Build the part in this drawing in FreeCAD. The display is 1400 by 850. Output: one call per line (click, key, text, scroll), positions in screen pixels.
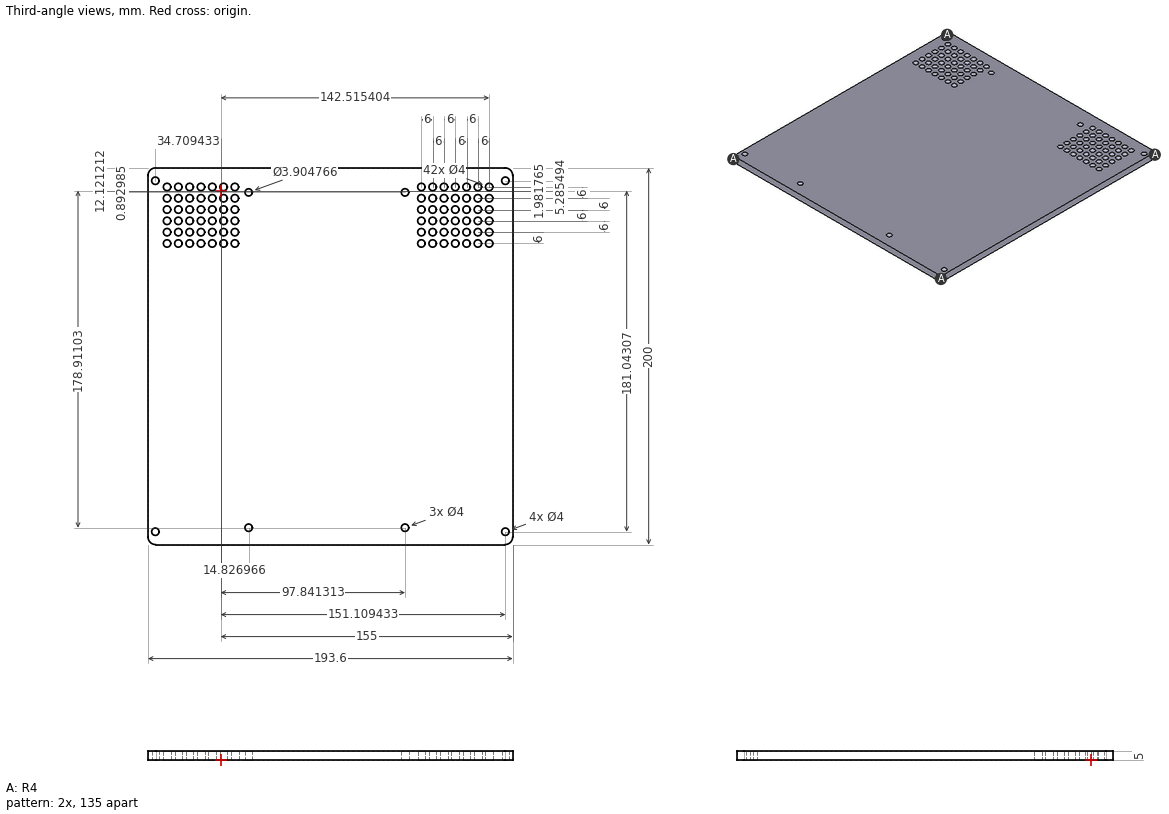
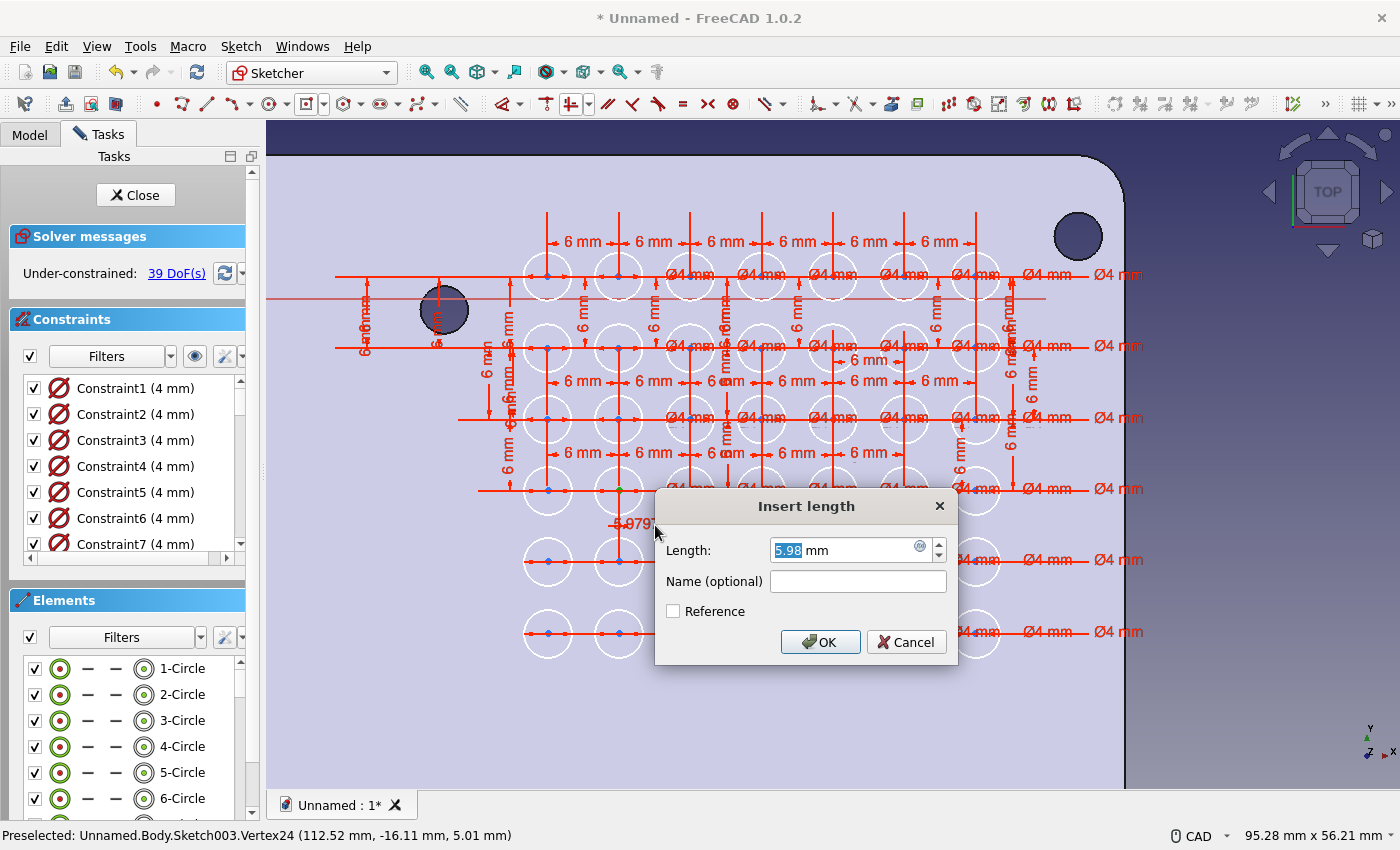
text(6)
key(Return)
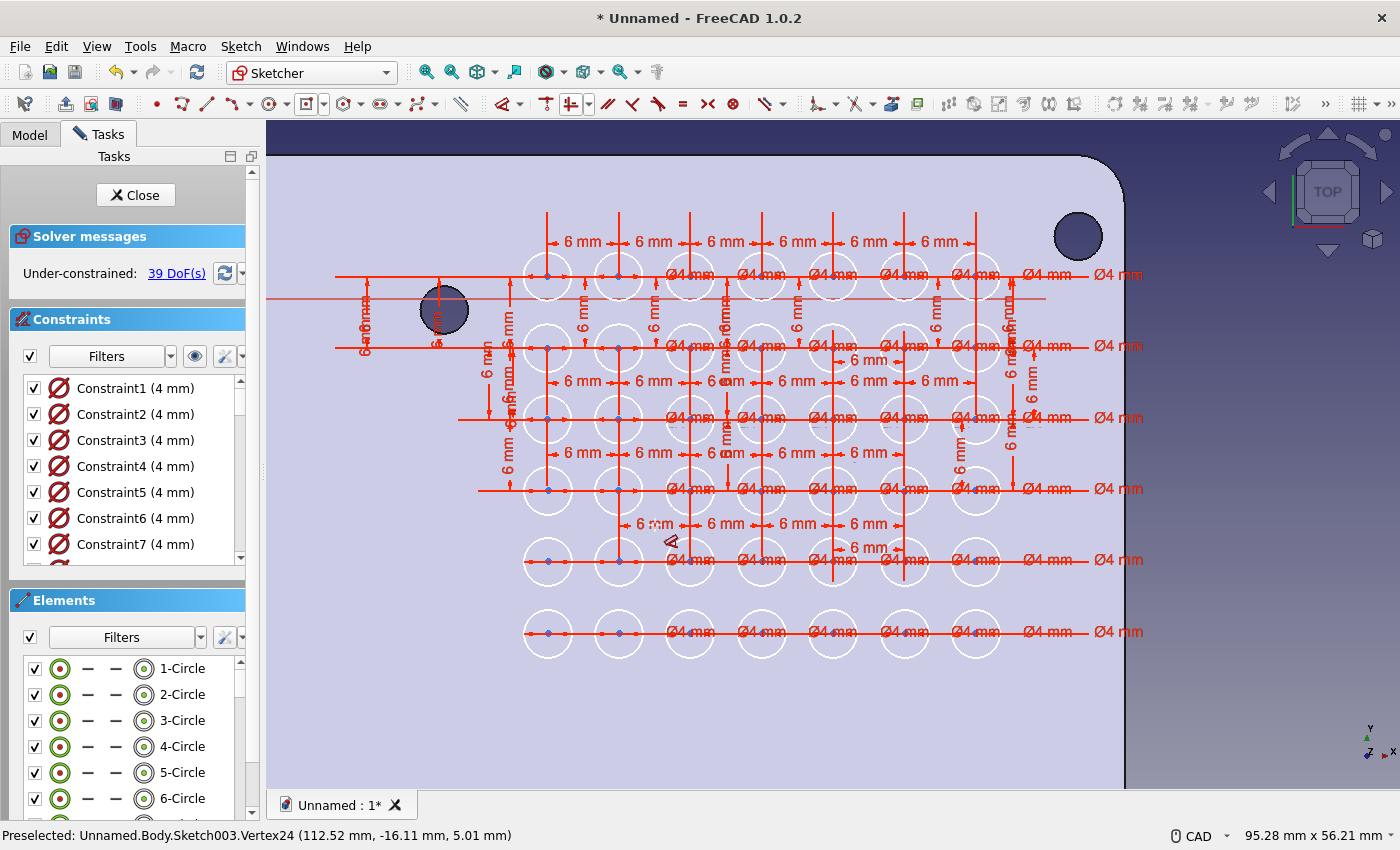
click(619, 420)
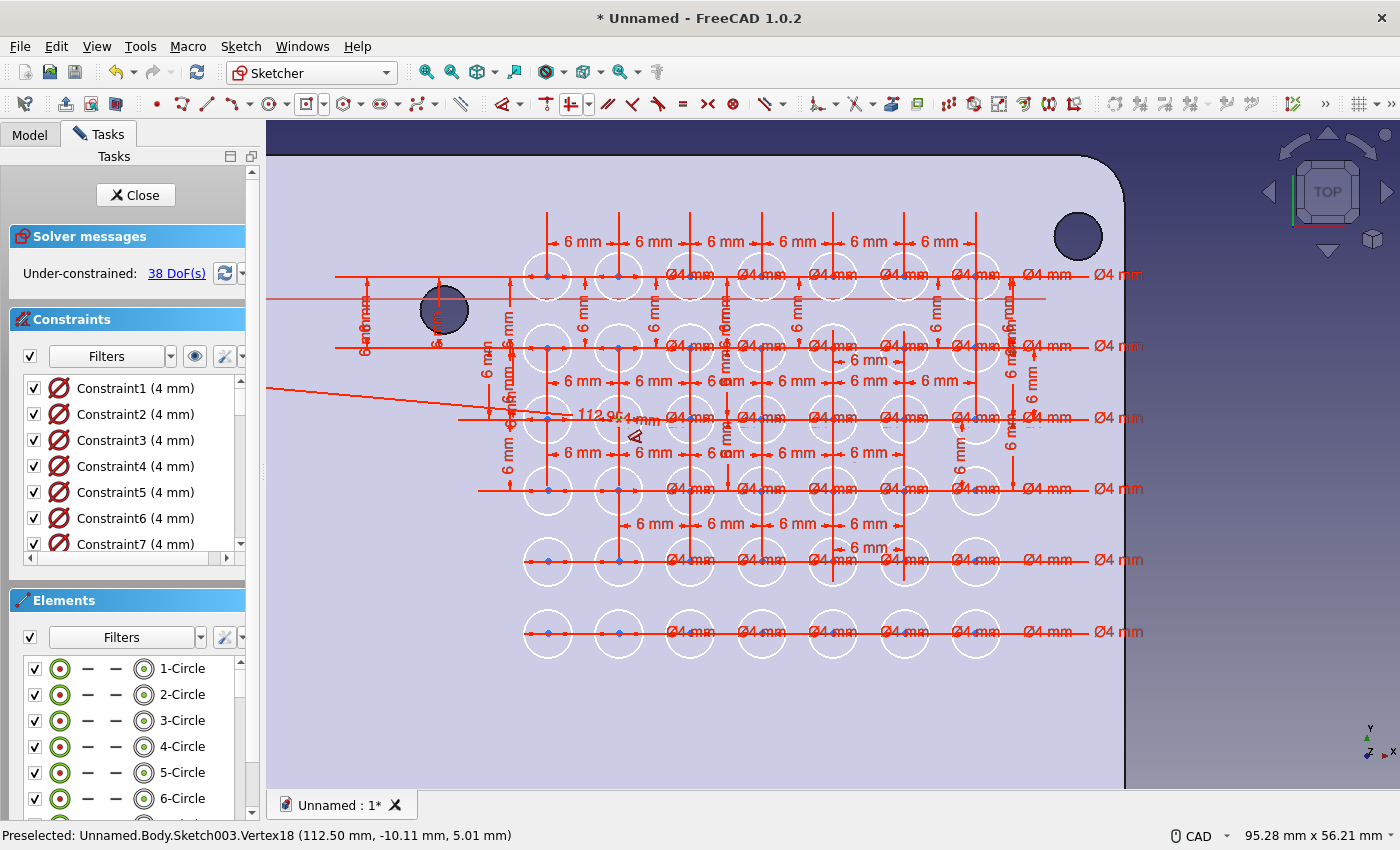
click(619, 491)
click(513, 480)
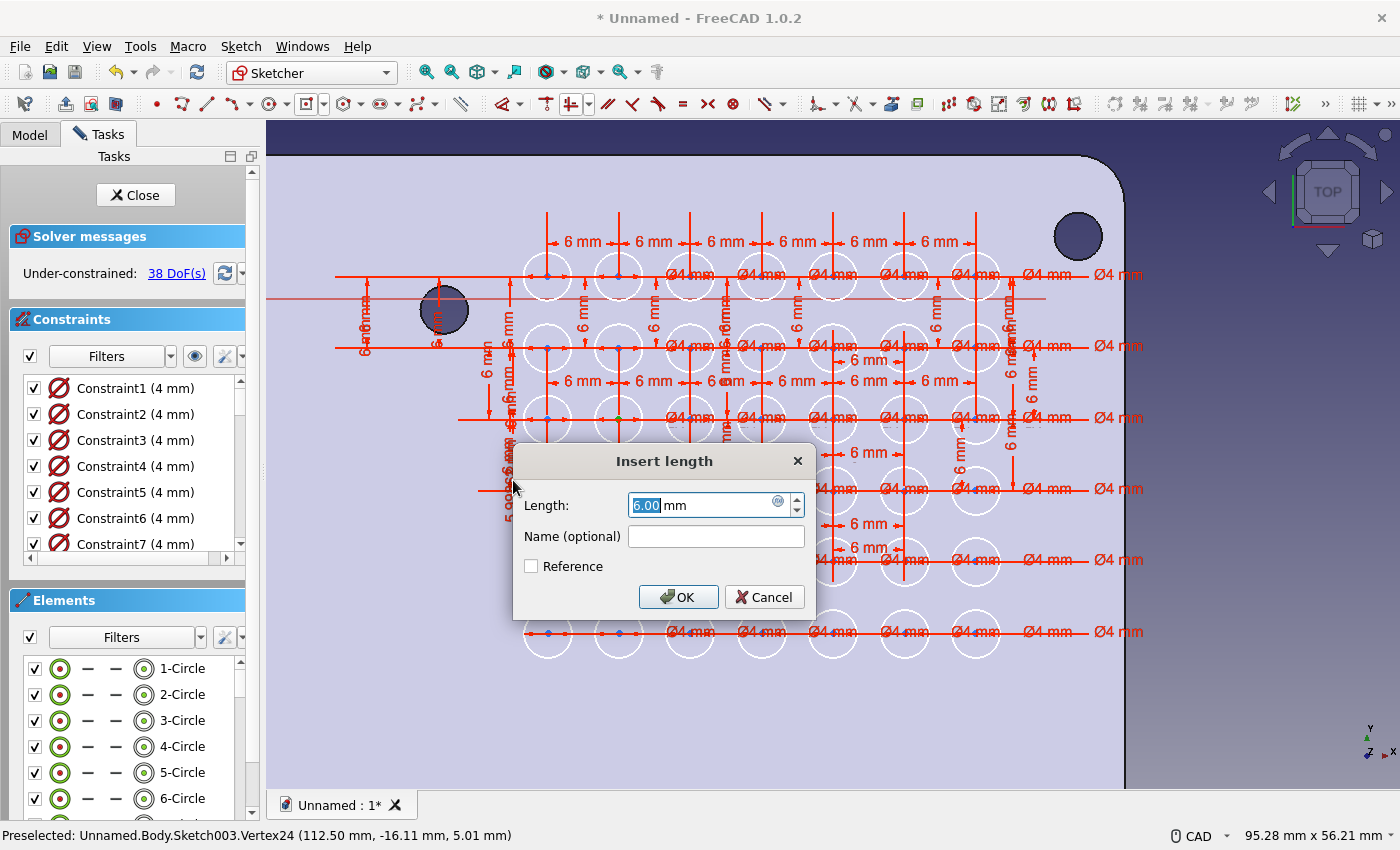
text(6)
key(Return)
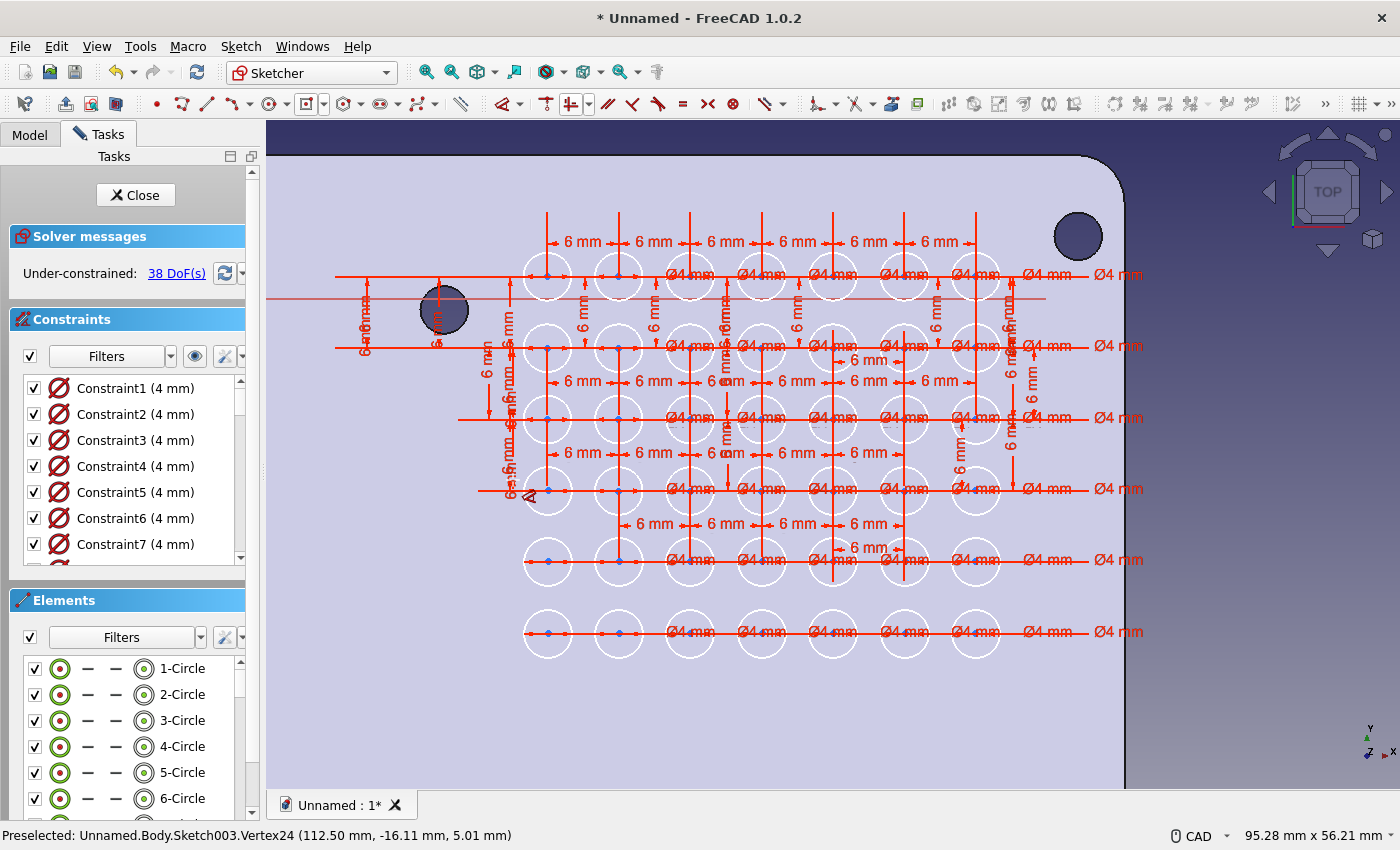
click(619, 491)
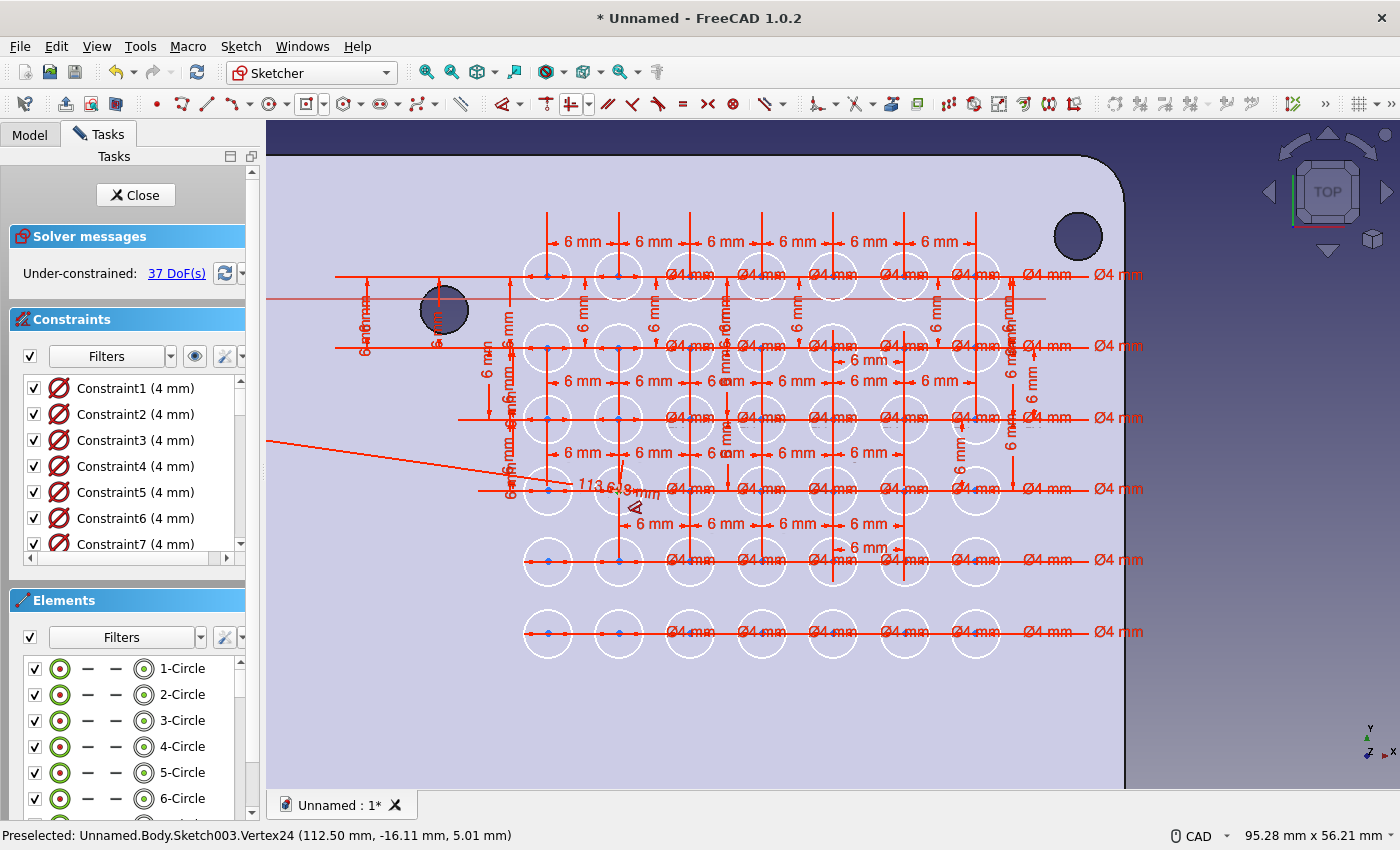
click(548, 491)
click(583, 525)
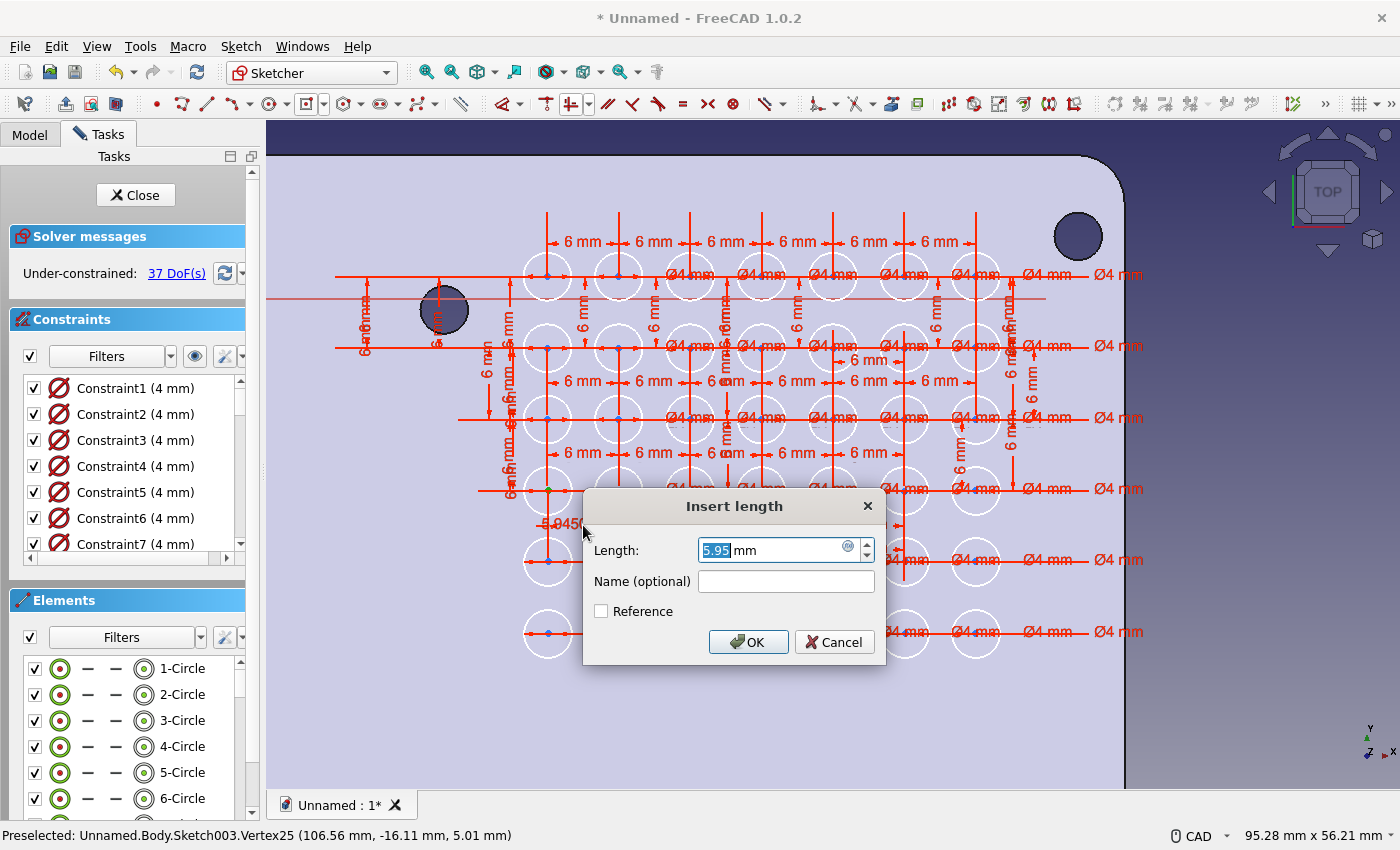
text(6)
key(Return)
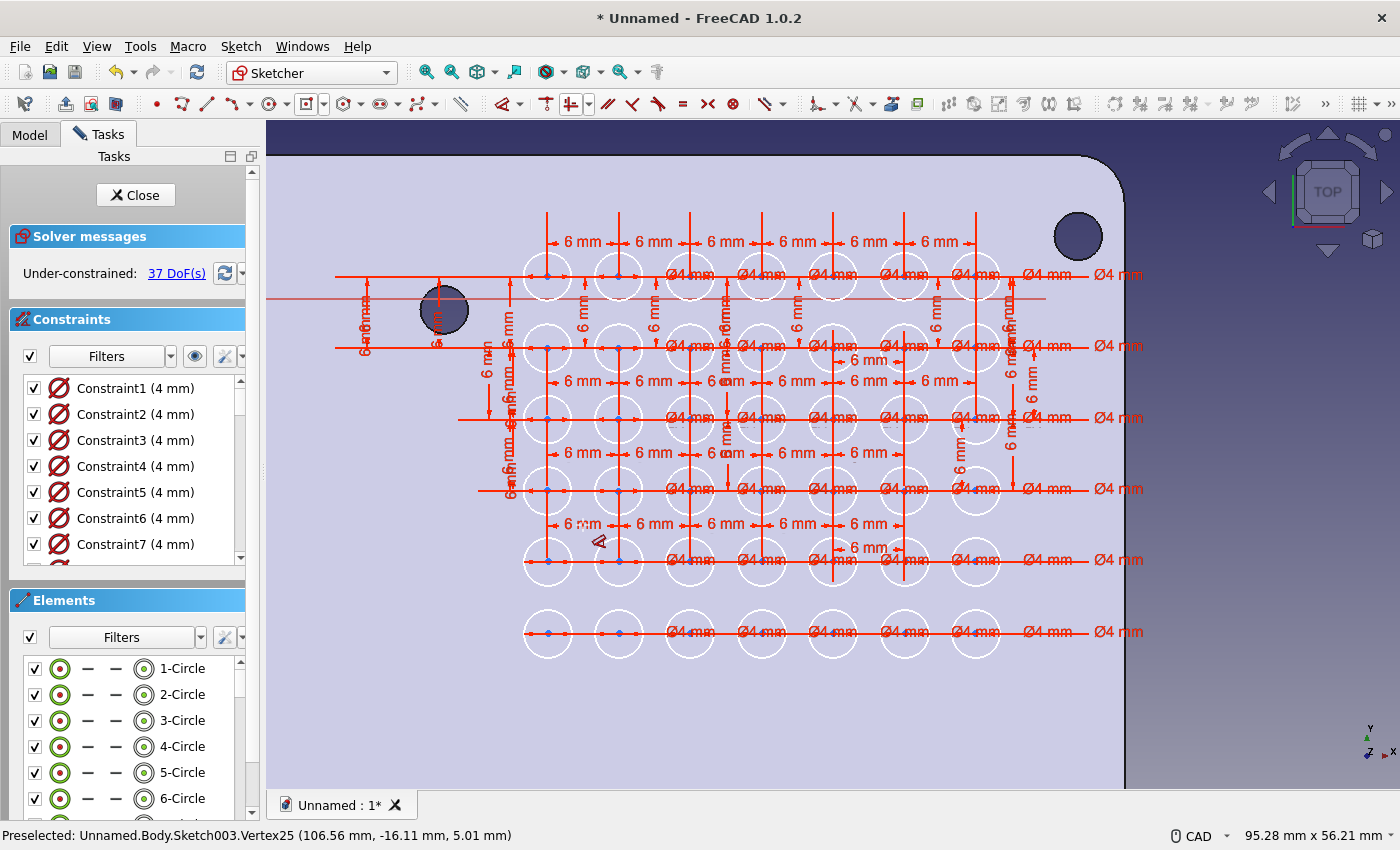
click(547, 420)